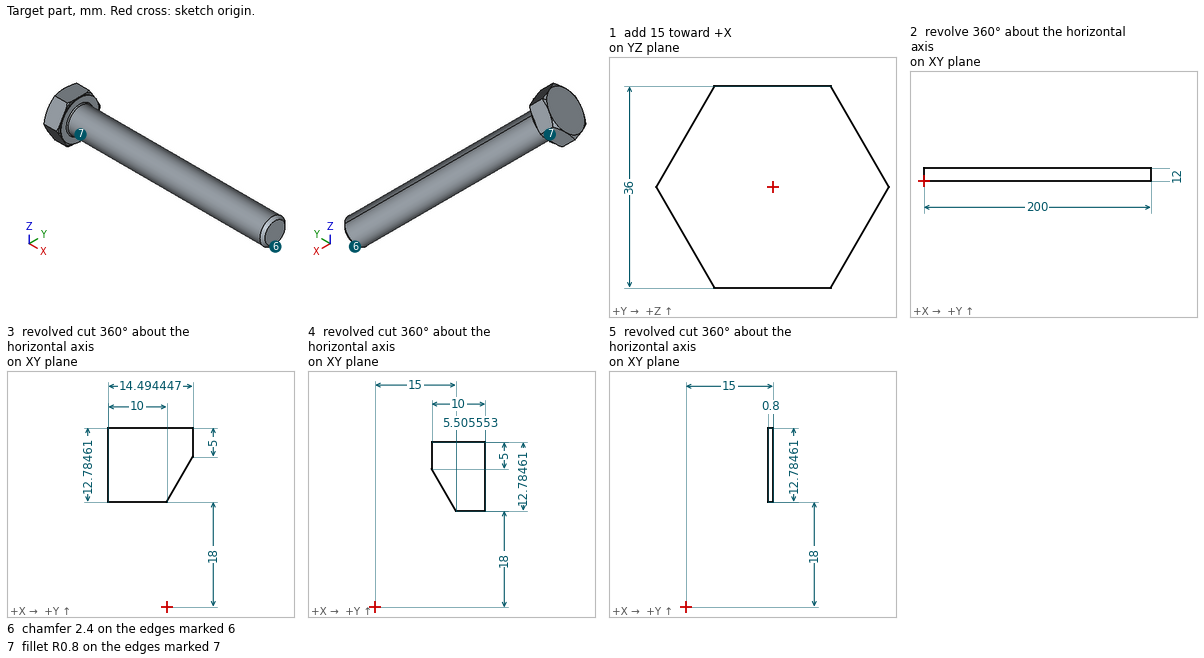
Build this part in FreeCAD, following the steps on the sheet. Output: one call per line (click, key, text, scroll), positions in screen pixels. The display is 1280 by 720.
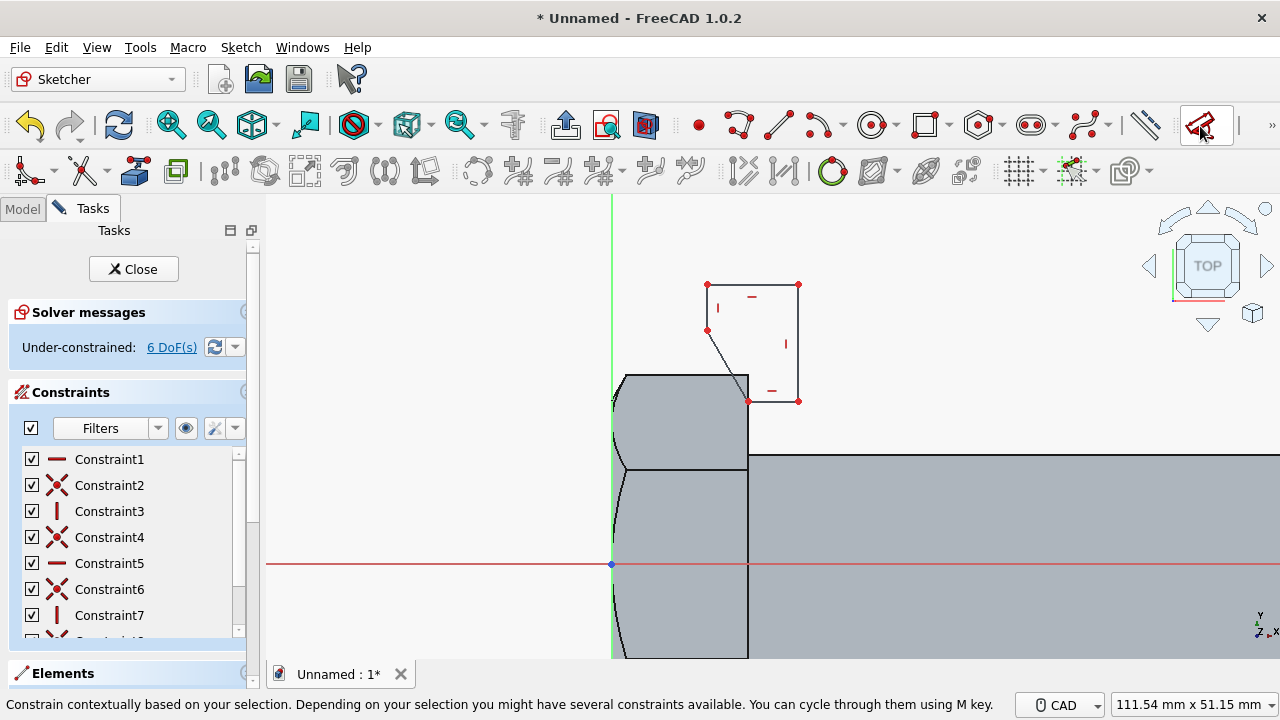
click(707, 299)
click(741, 308)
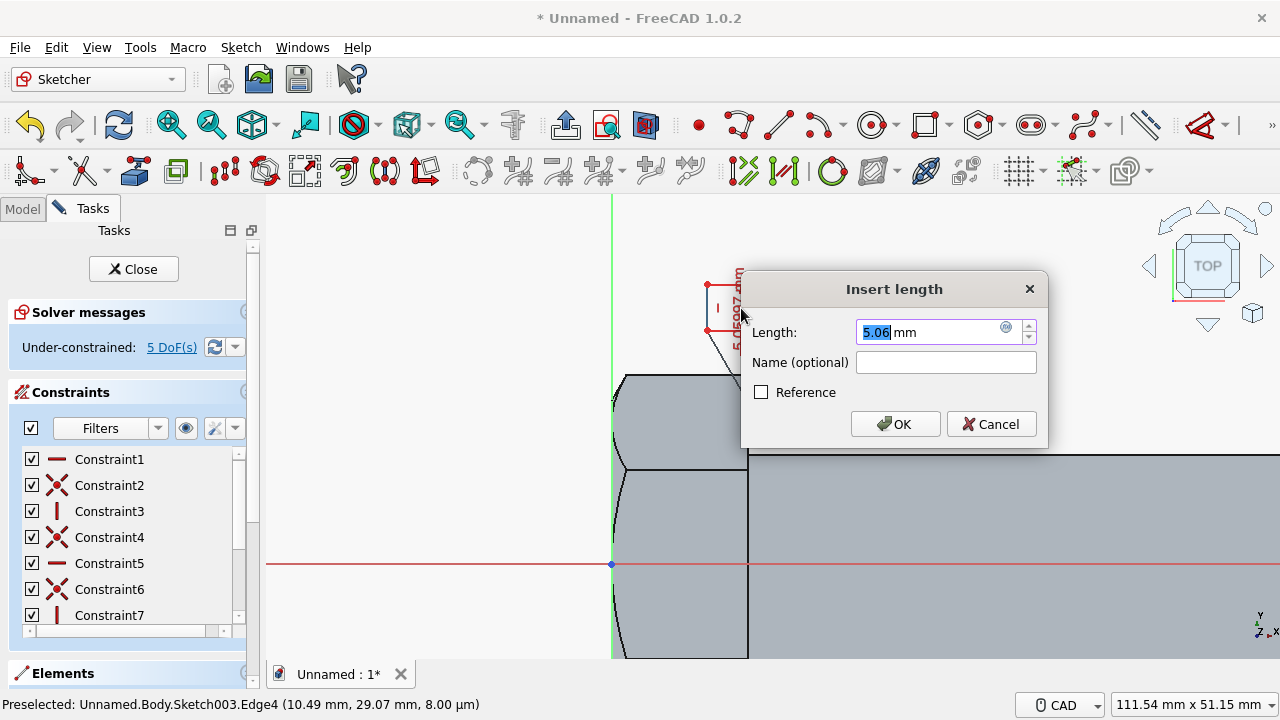
text(5)
key(Return)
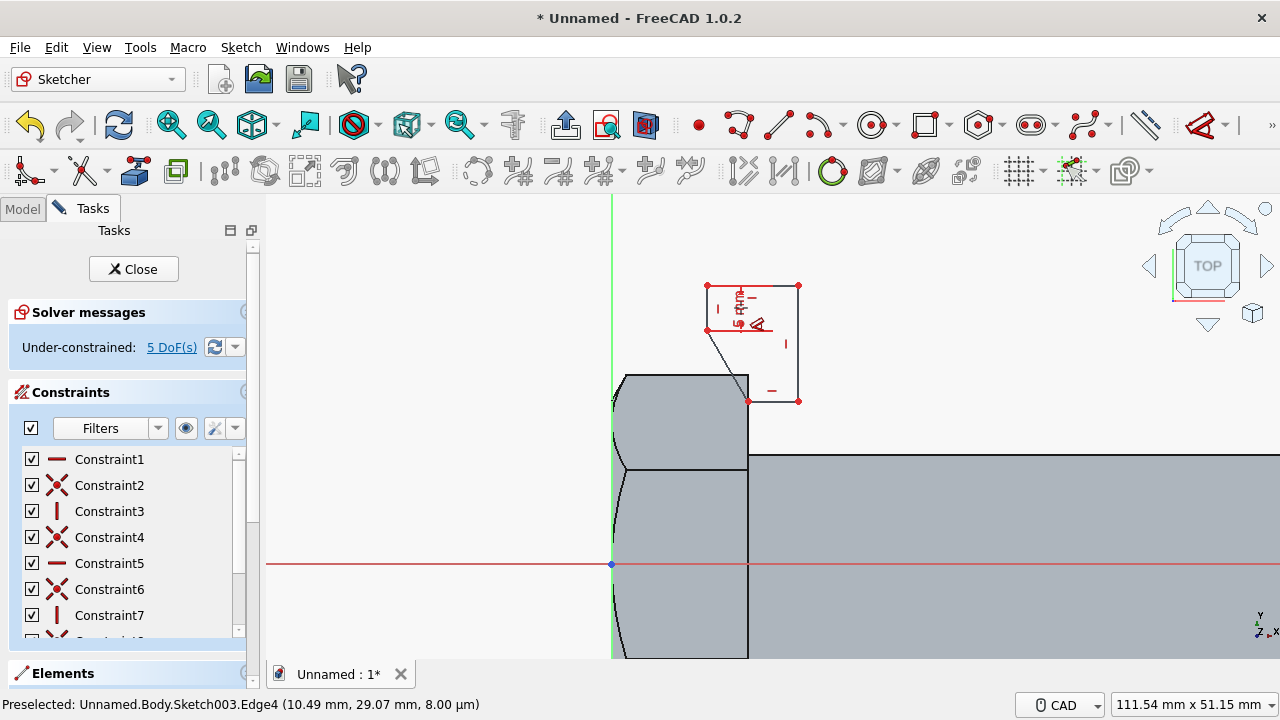
click(771, 286)
click(752, 252)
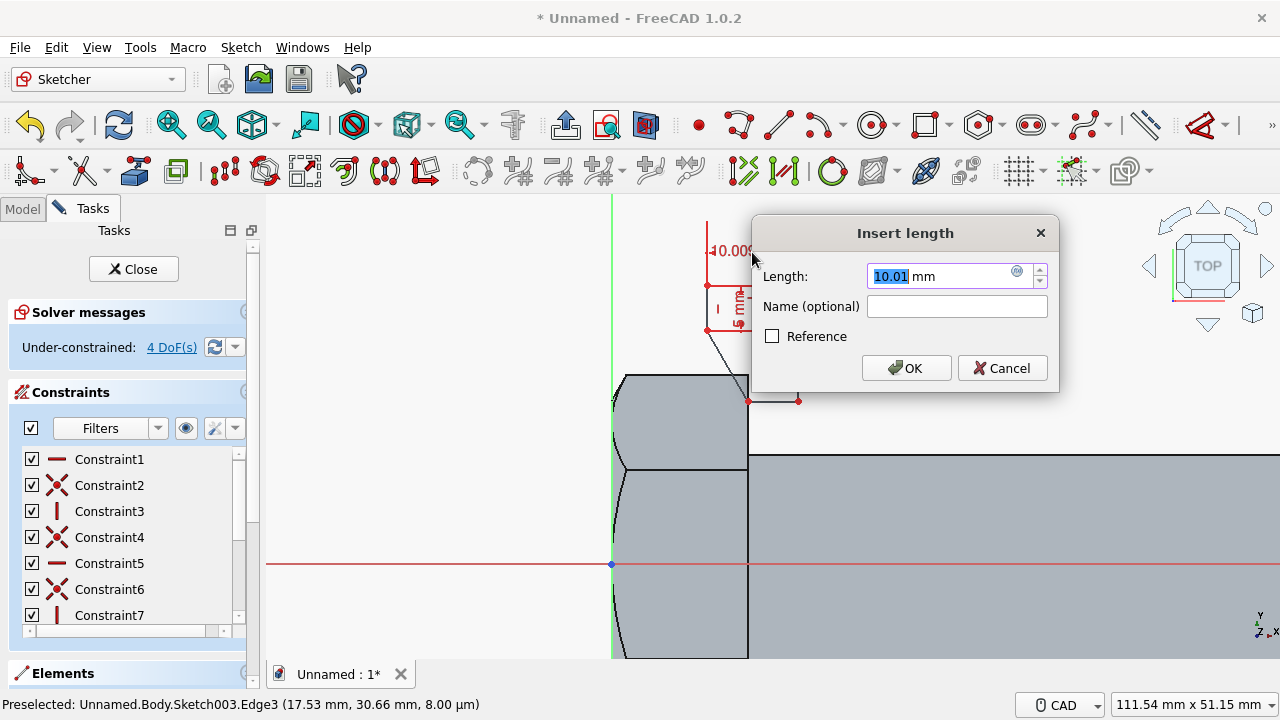
text(10)
key(Return)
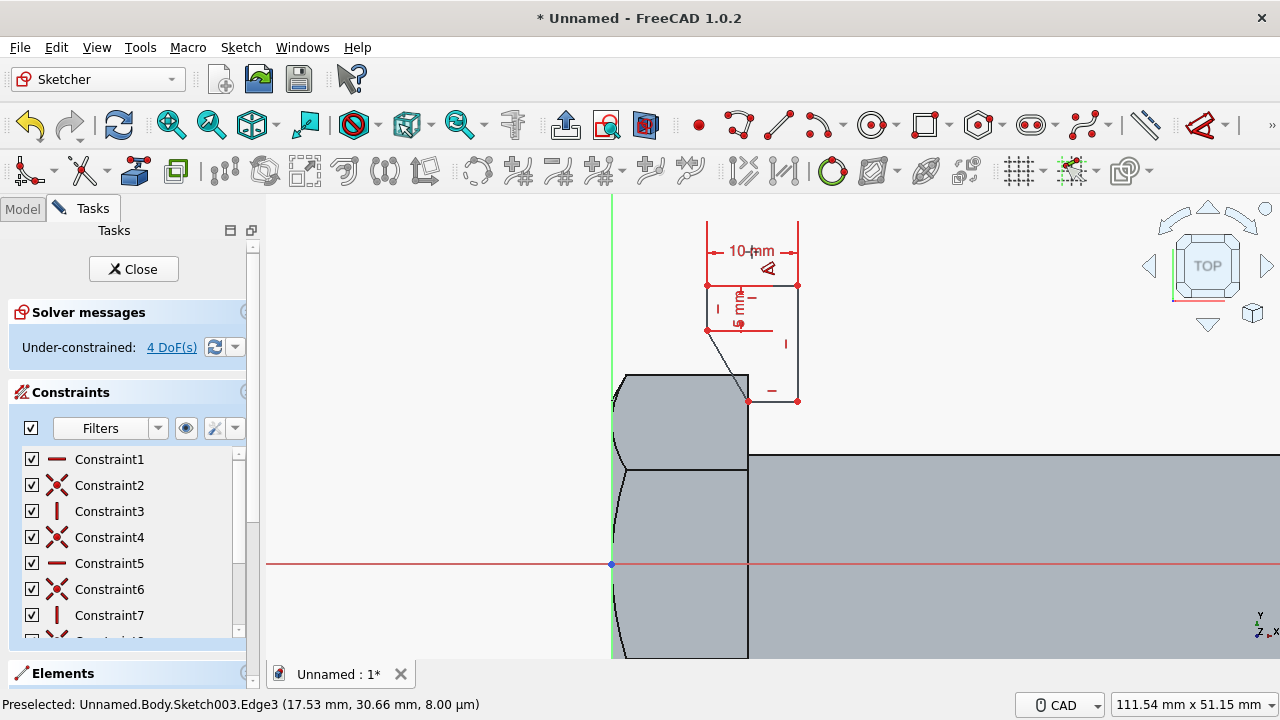
click(748, 402)
click(680, 598)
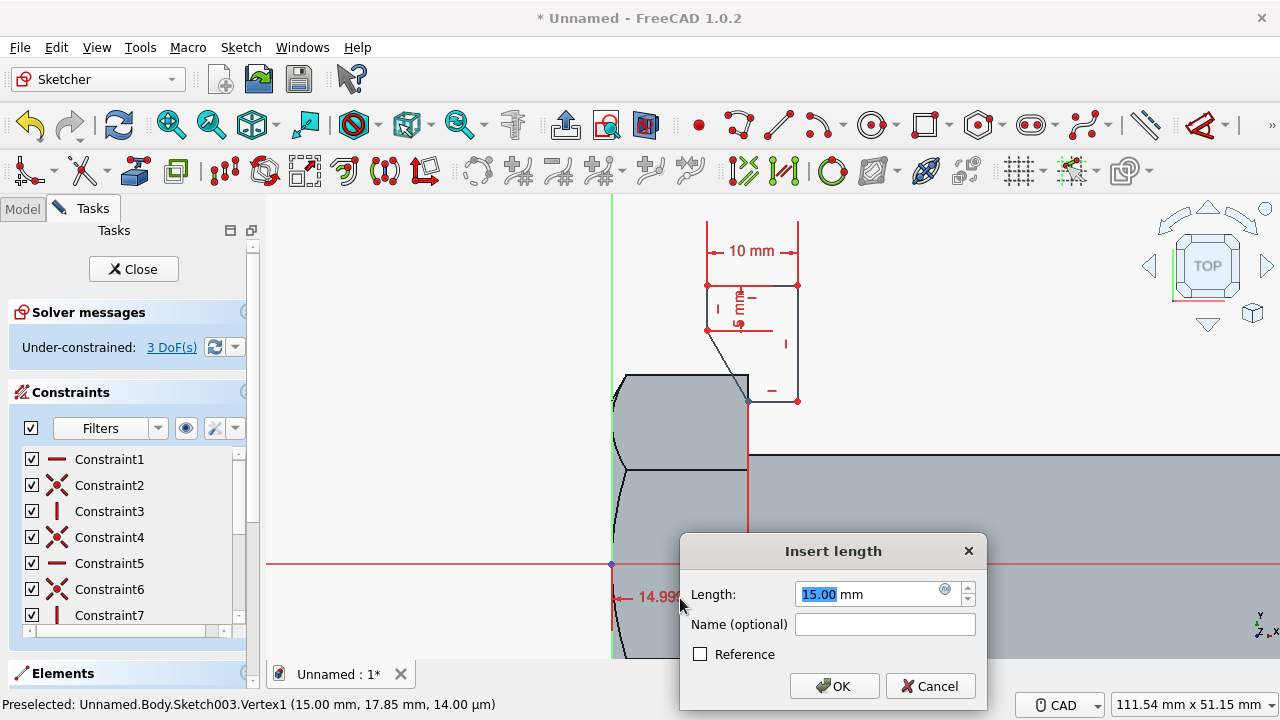
text(15)
key(Return)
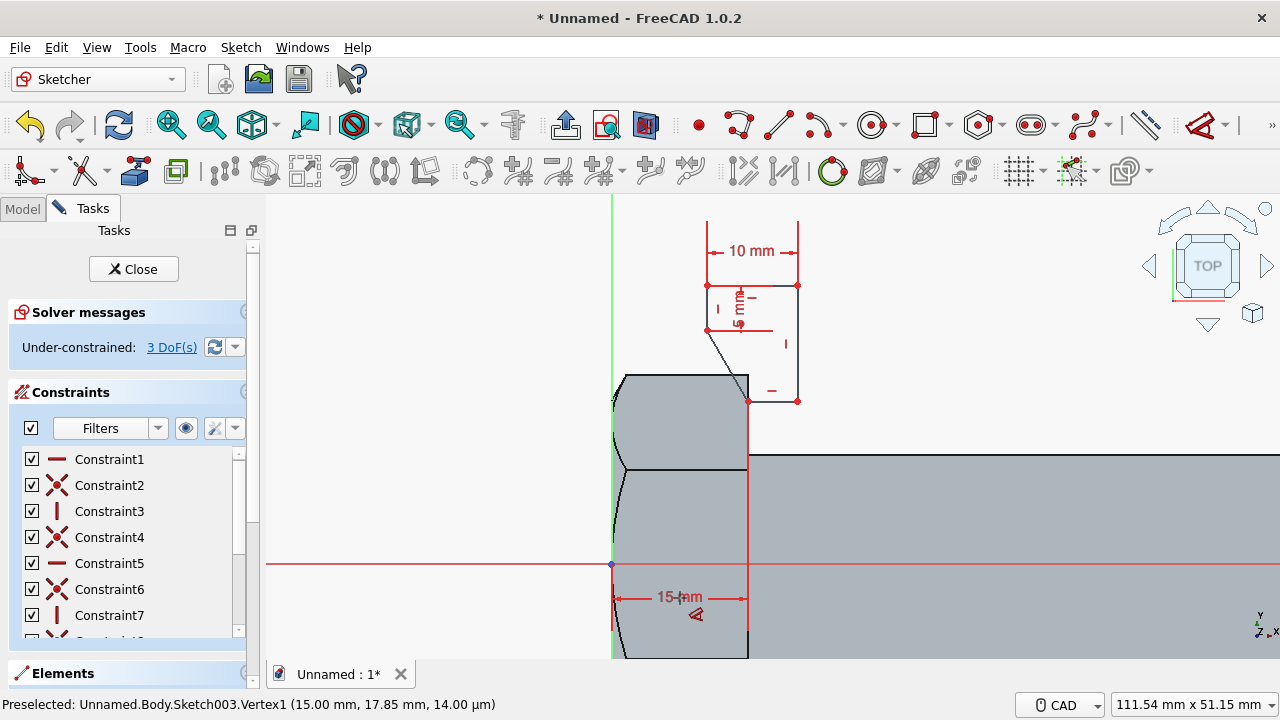
click(748, 402)
click(578, 483)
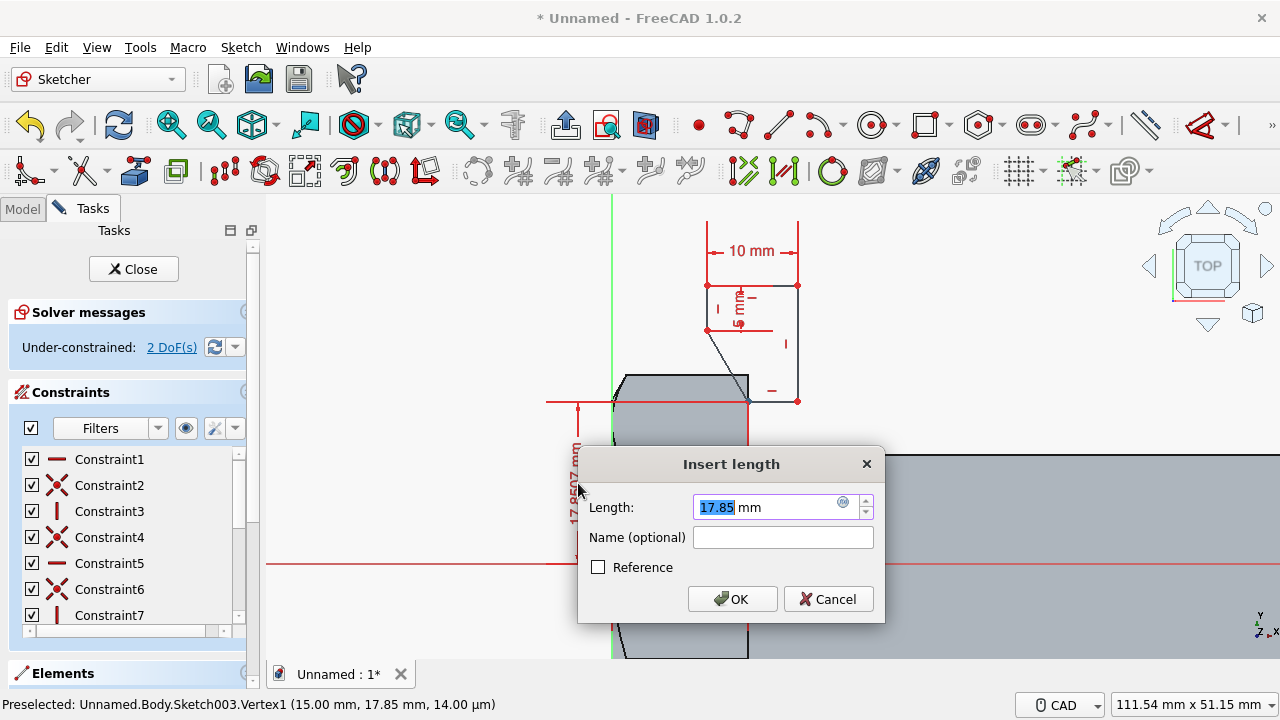
text(18)
key(Return)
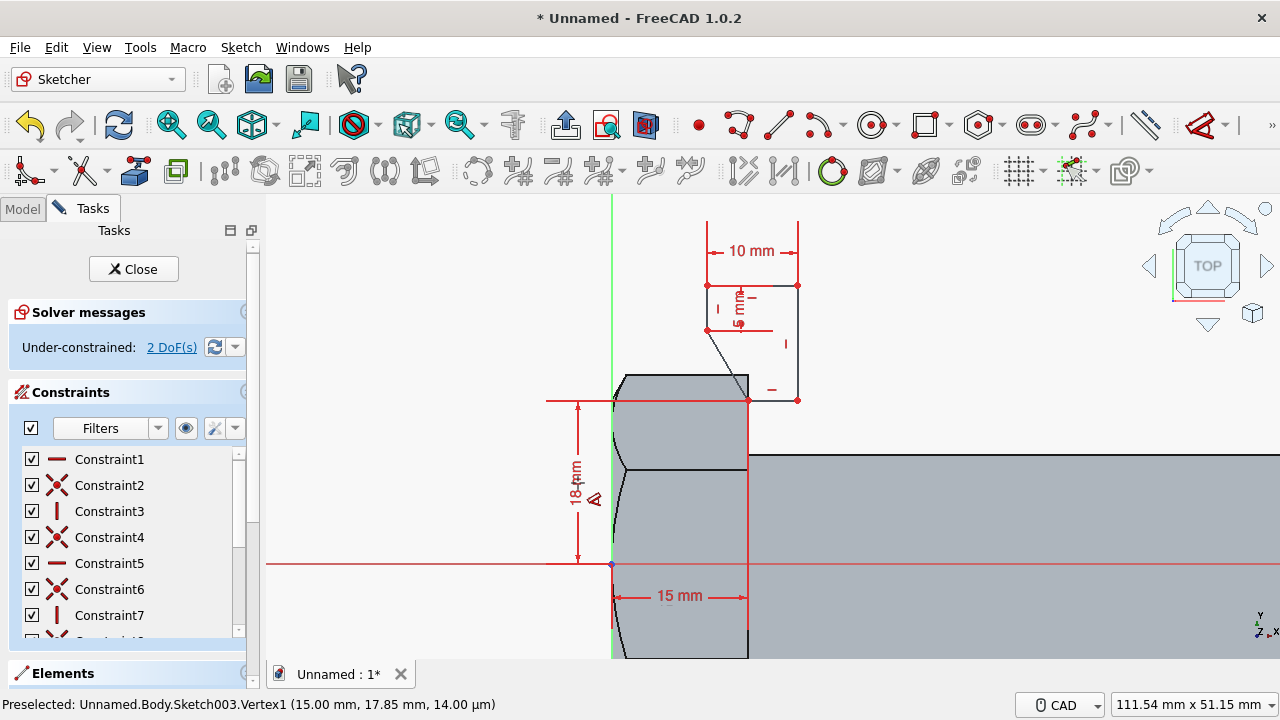
click(763, 401)
click(773, 367)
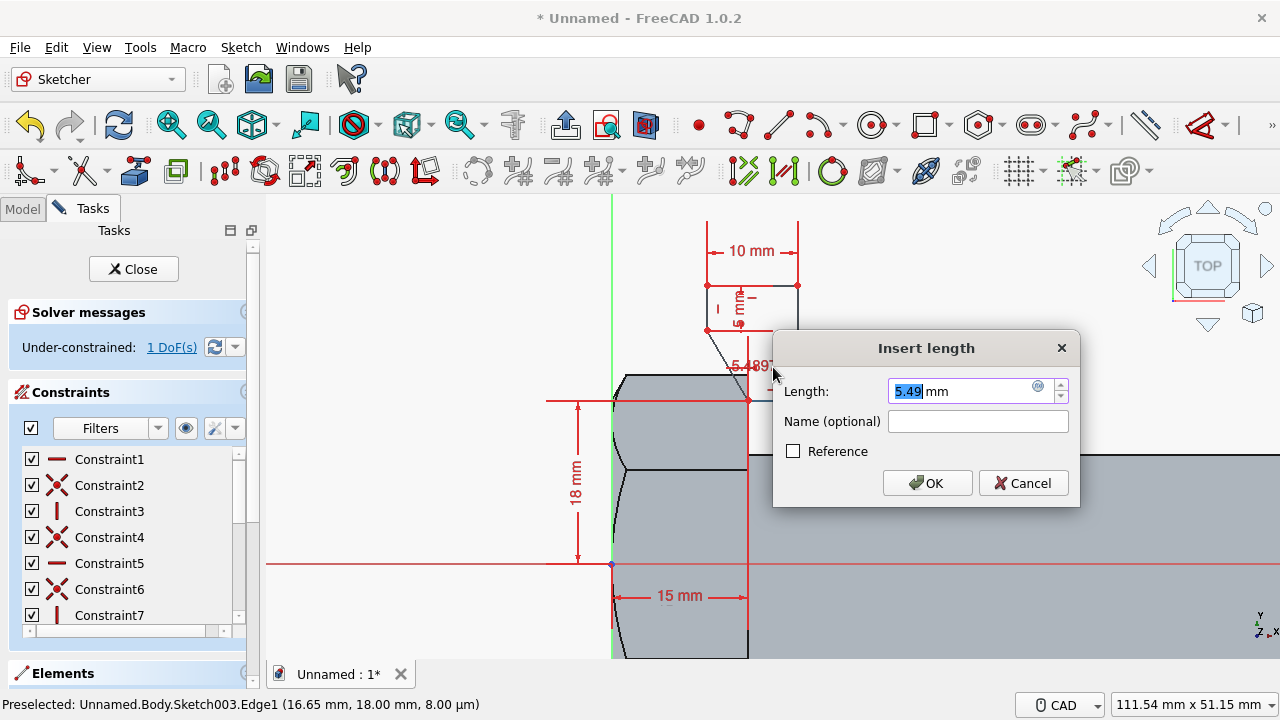
text(5.505553)
key(Return)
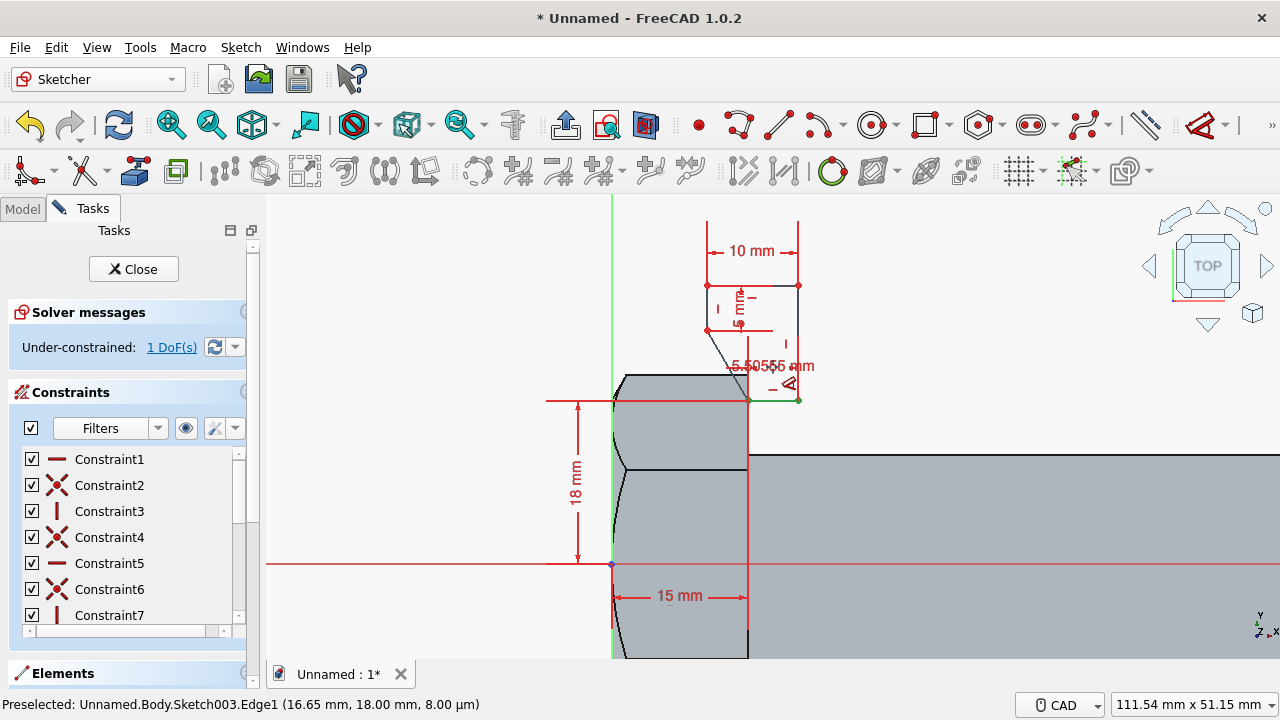
click(798, 366)
click(832, 343)